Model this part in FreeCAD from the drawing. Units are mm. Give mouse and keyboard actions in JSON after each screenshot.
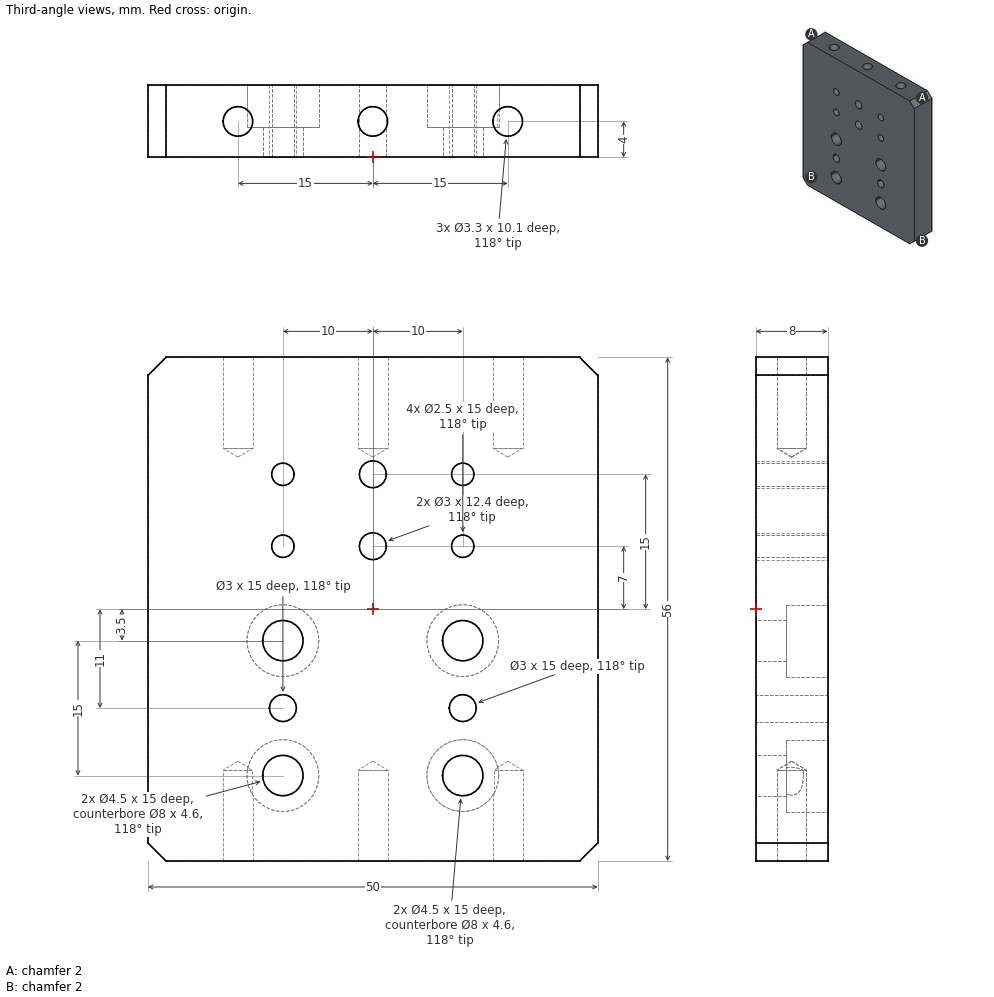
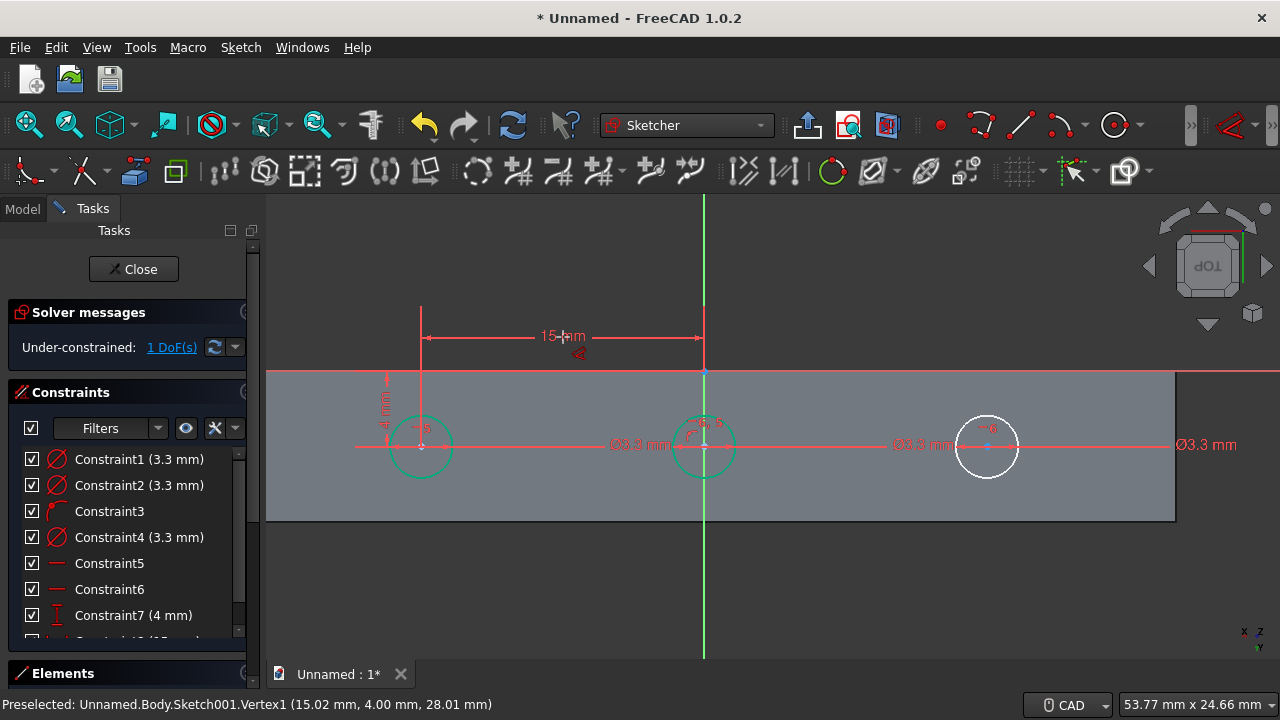
{"action": "left_click", "coordinate": [987, 447]}
{"action": "left_click", "coordinate": [846, 337]}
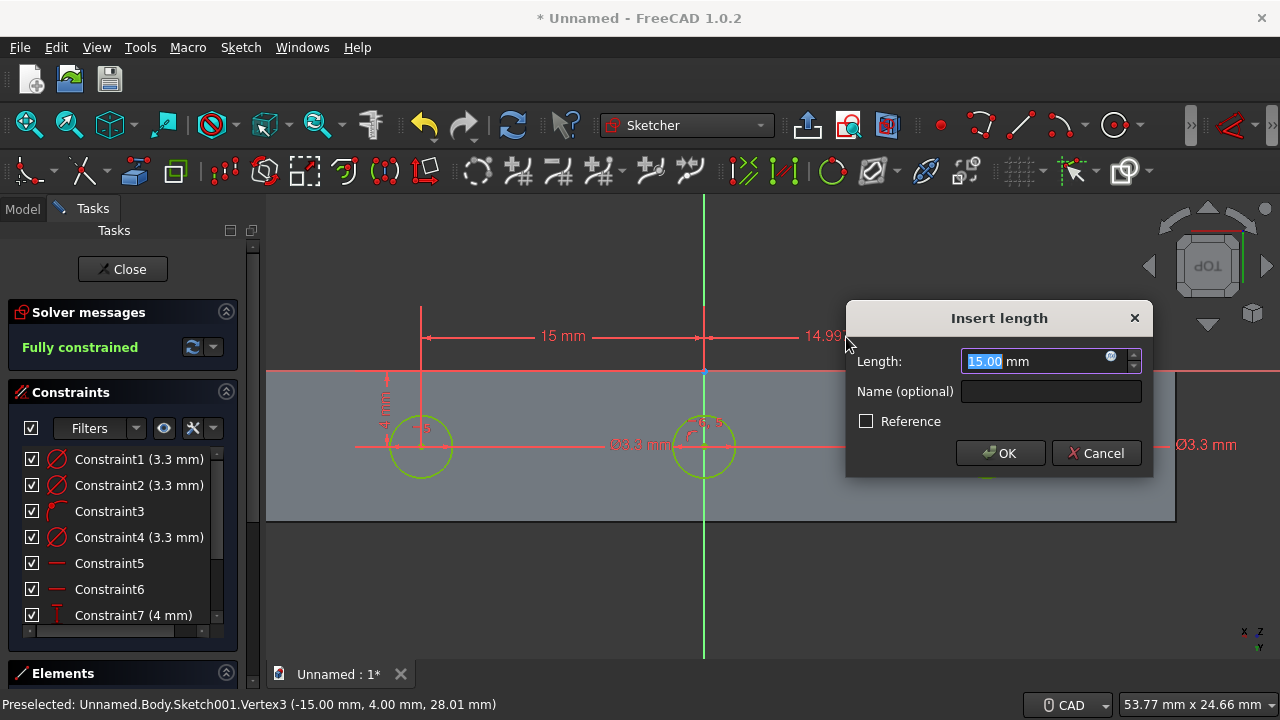
{"action": "type", "text": "15"}
{"action": "key", "text": "Return"}
{"action": "key", "text": "Escape"}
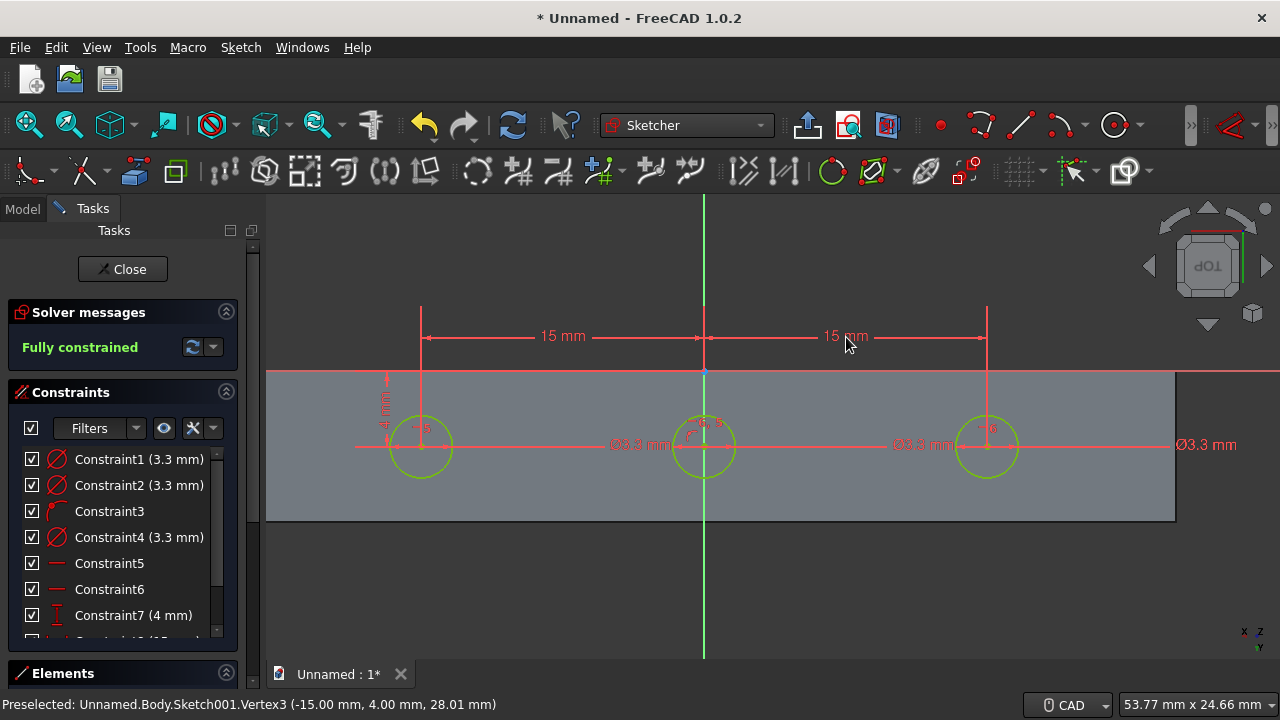
{"action": "left_click", "coordinate": [123, 269]}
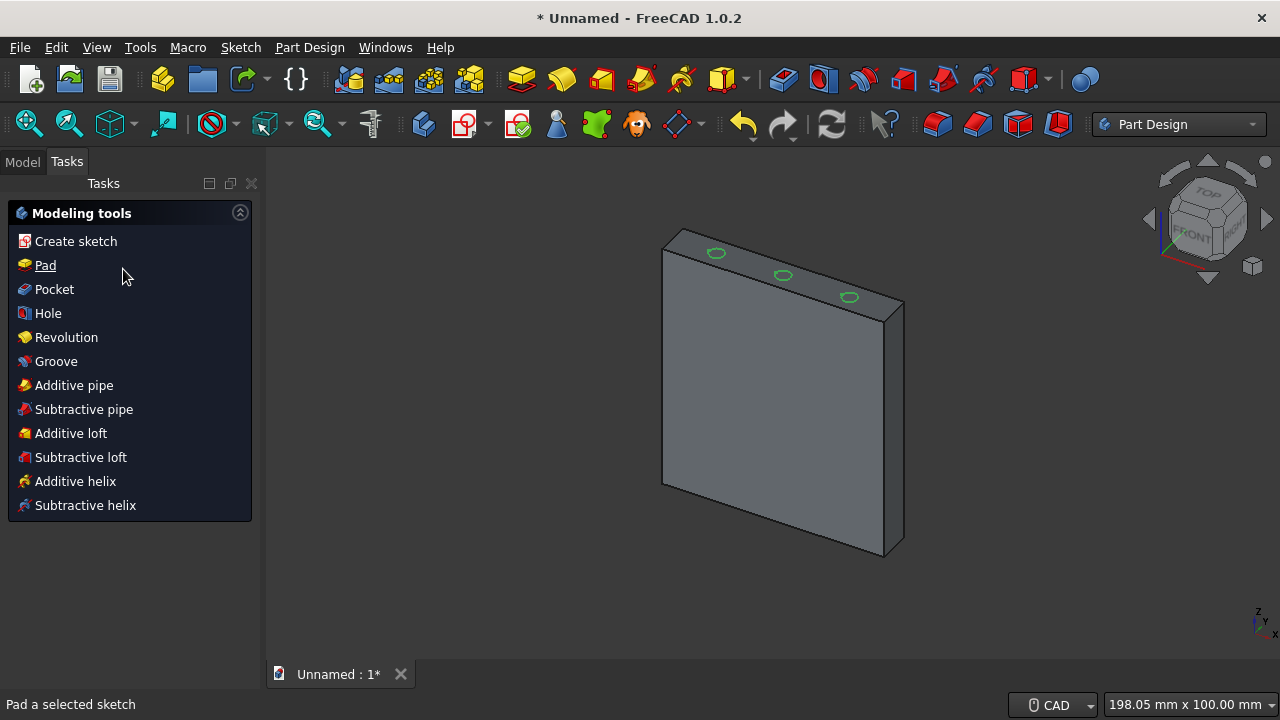
{"action": "left_click", "coordinate": [824, 80]}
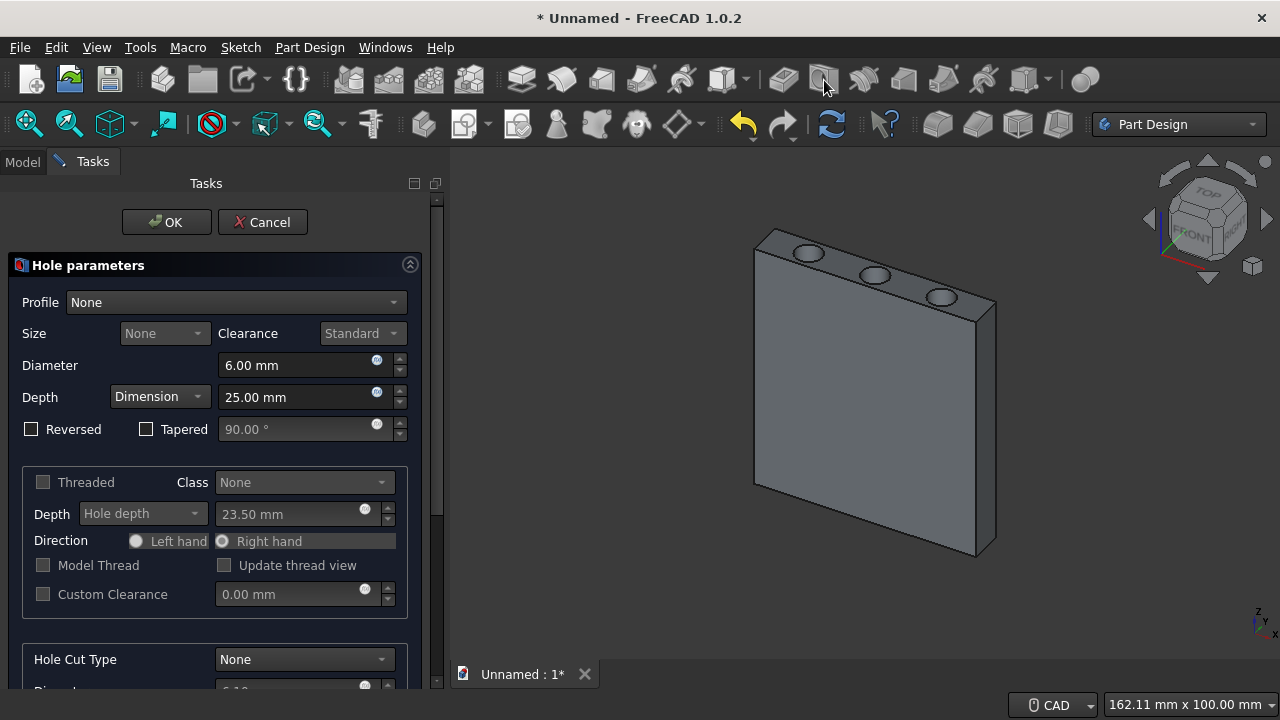
{"action": "triple_click", "coordinate": [305, 365]}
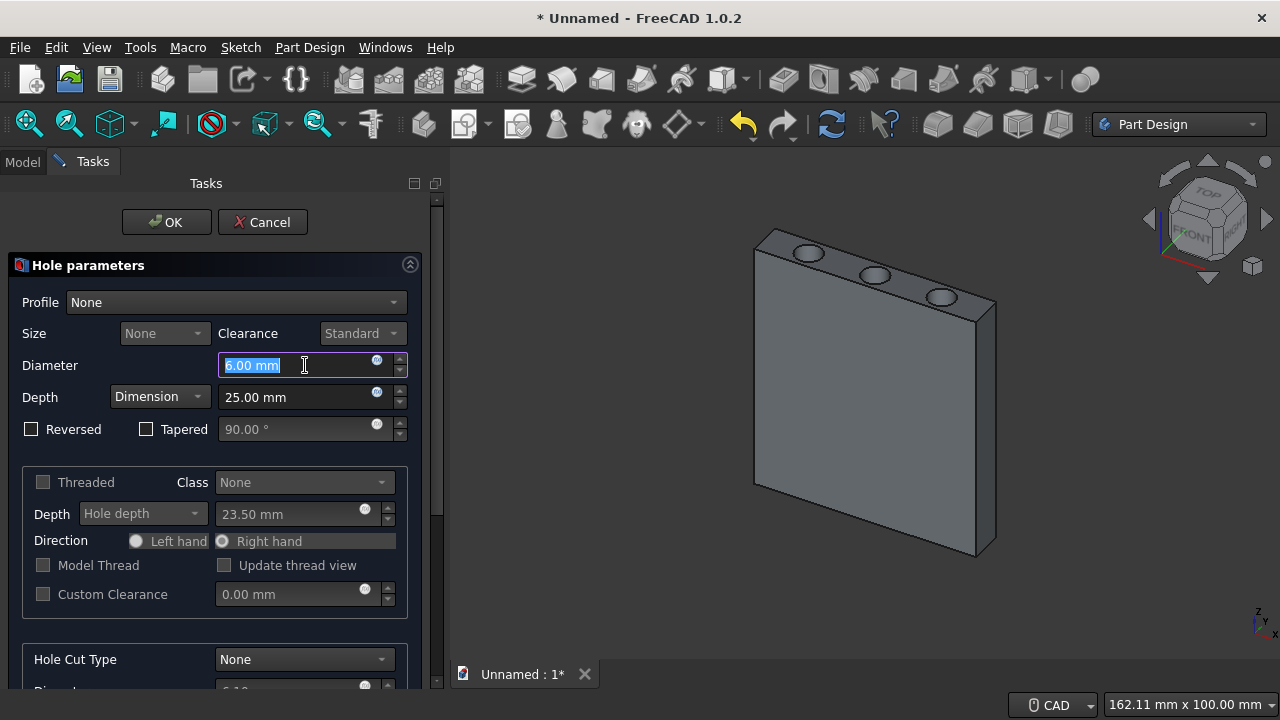
{"action": "type", "text": "3.3"}
{"action": "key", "text": "Tab"}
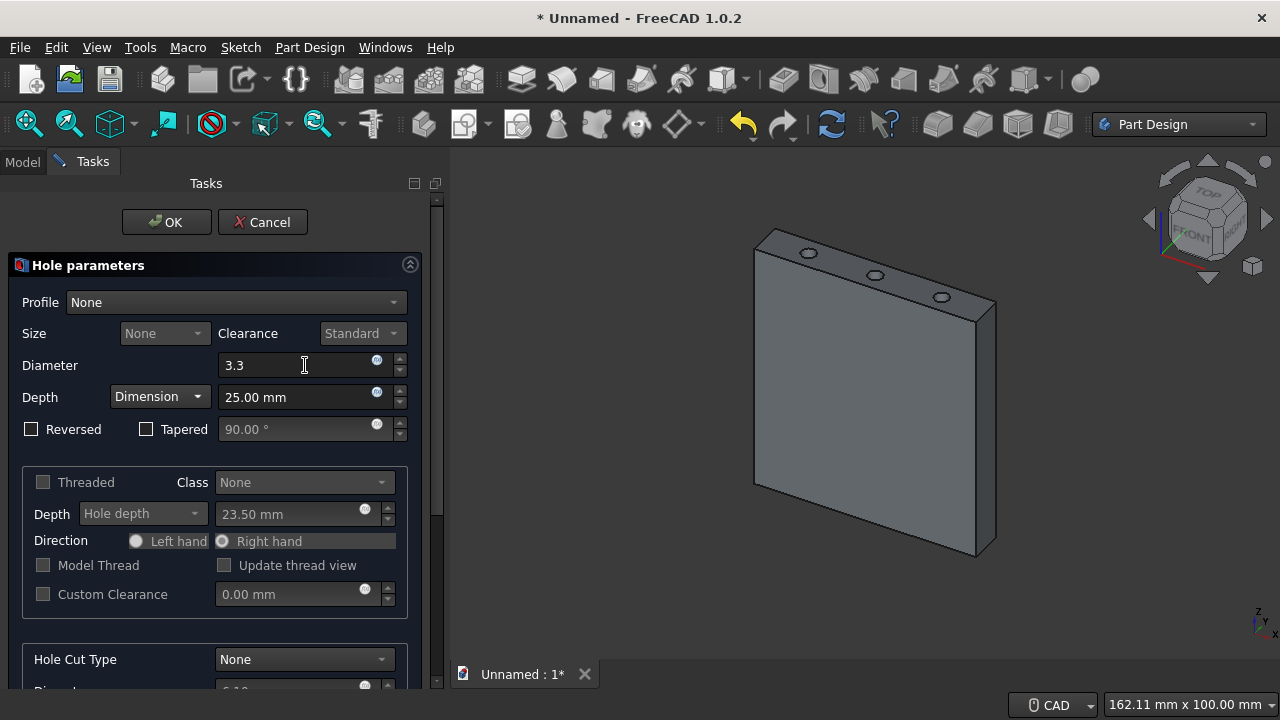
{"action": "triple_click", "coordinate": [305, 397]}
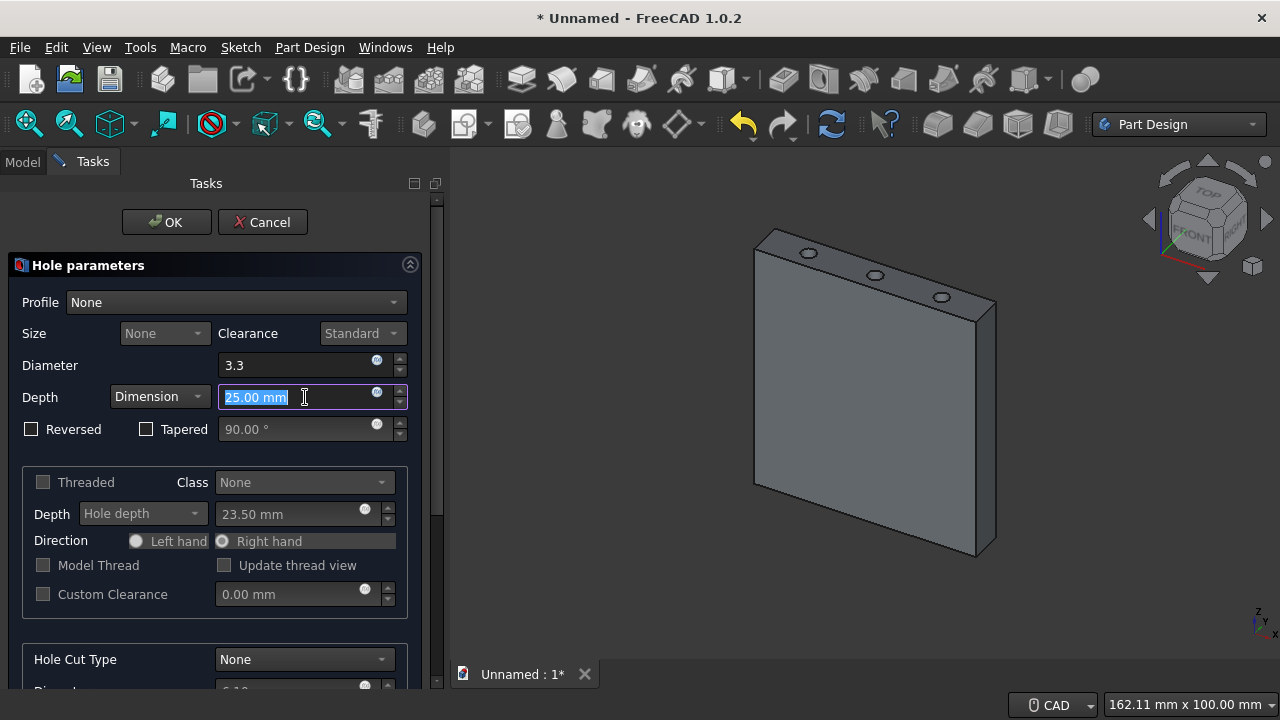
{"action": "type", "text": "10.1"}
{"action": "key", "text": "Tab"}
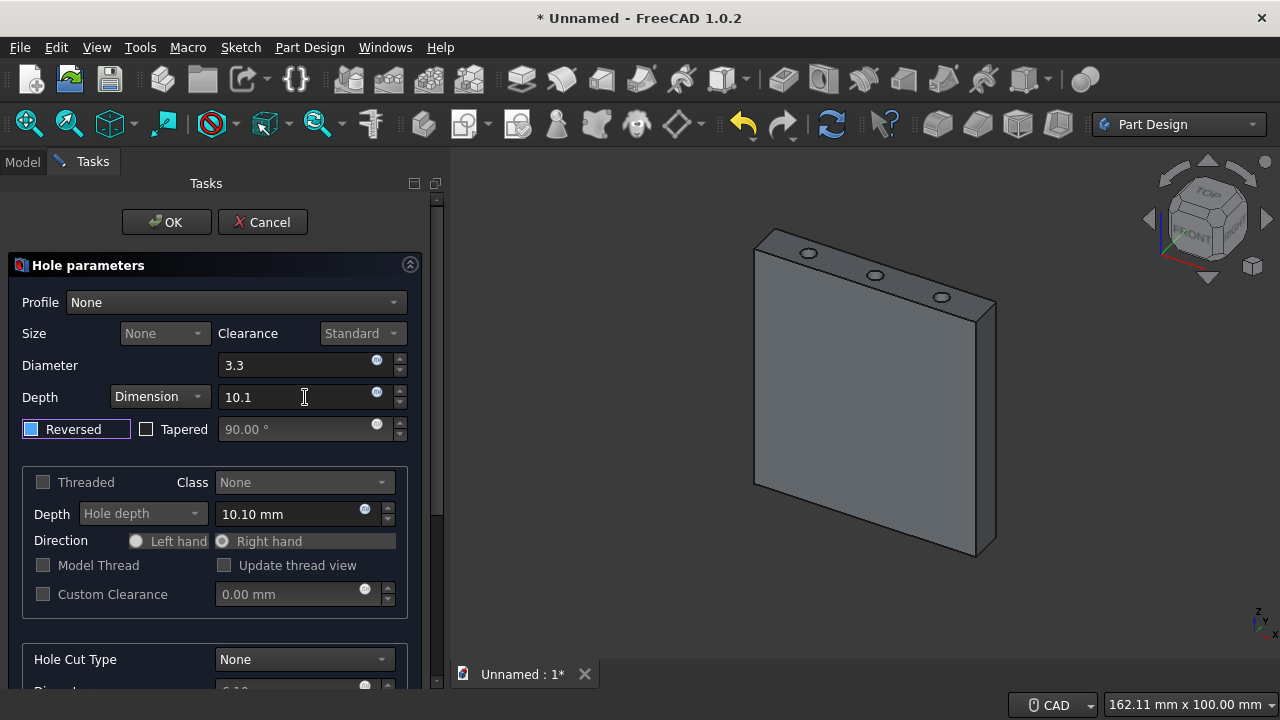
{"action": "left_click", "coordinate": [167, 222]}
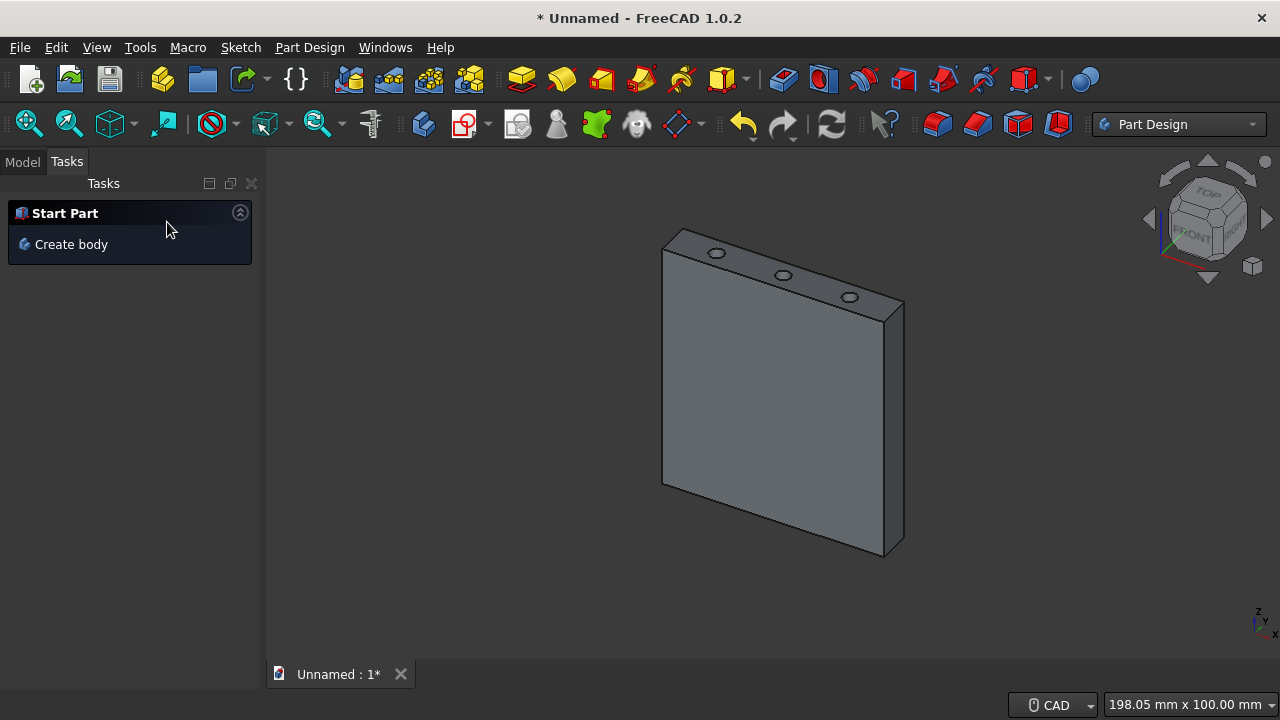
{"action": "left_click", "coordinate": [894, 311]}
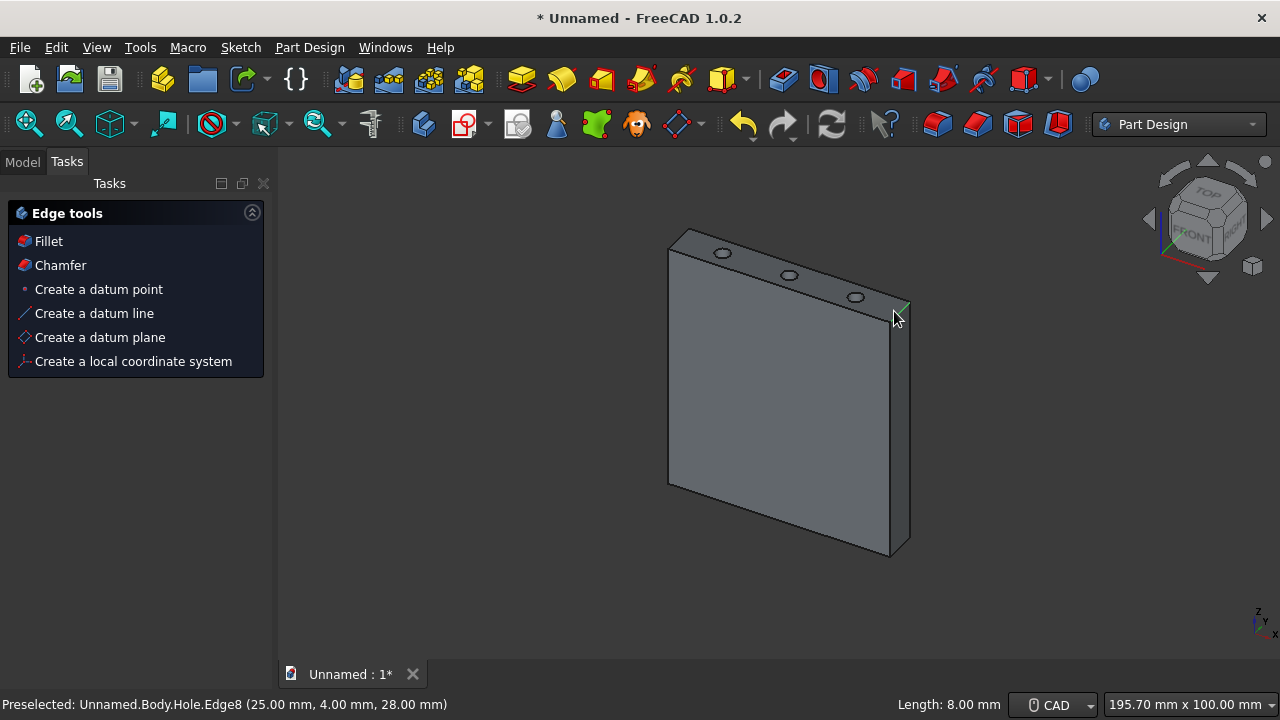
{"action": "key", "text": "0"}